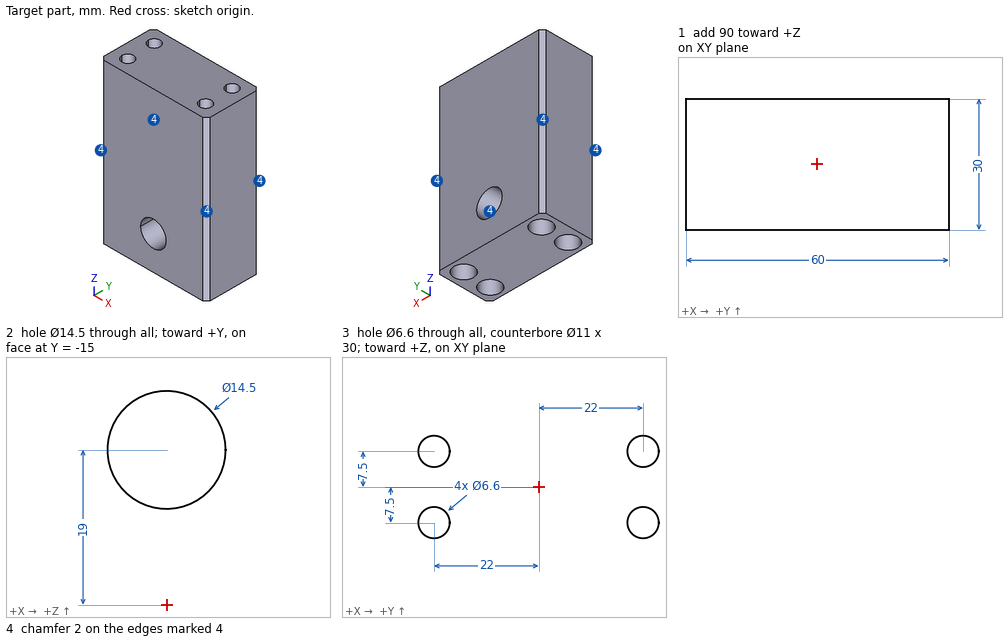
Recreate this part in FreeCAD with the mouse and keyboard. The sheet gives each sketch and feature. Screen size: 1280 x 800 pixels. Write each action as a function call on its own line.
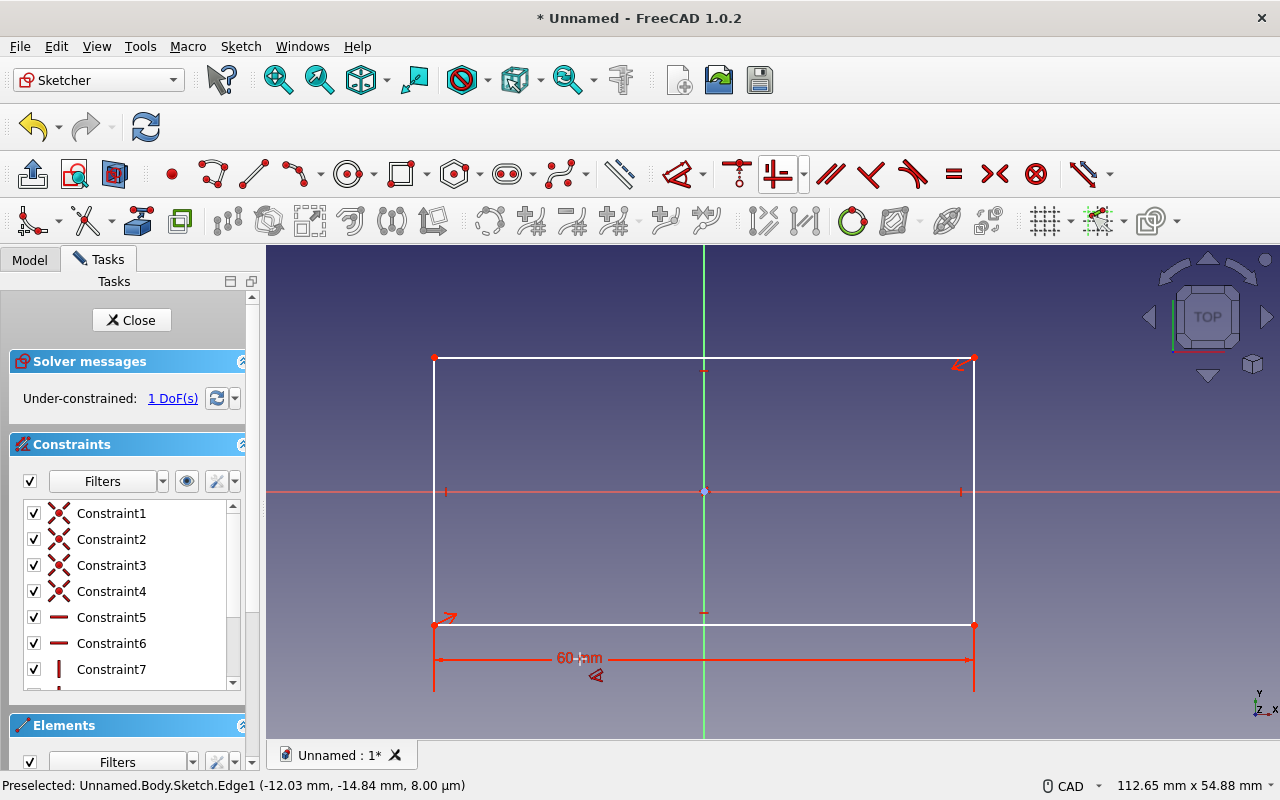
click(974, 545)
click(1008, 430)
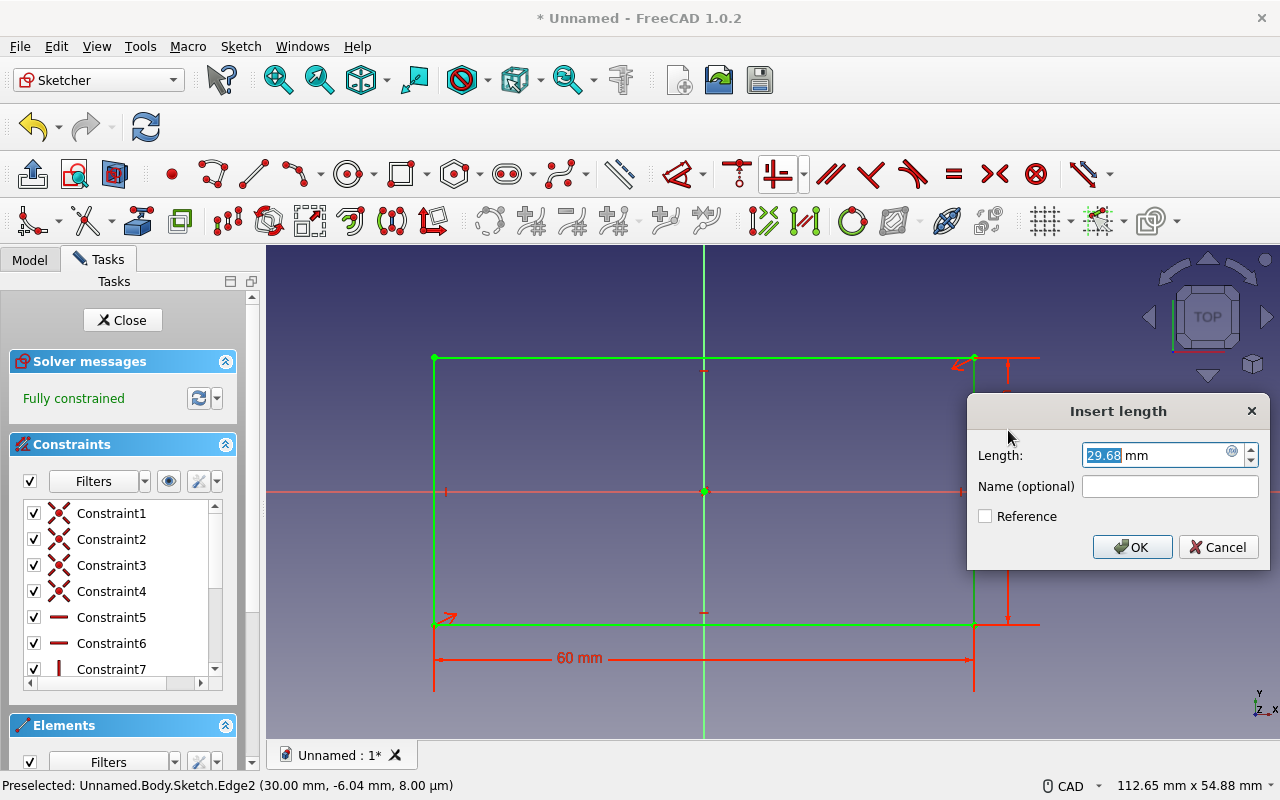
text(30)
key(Return)
key(Escape)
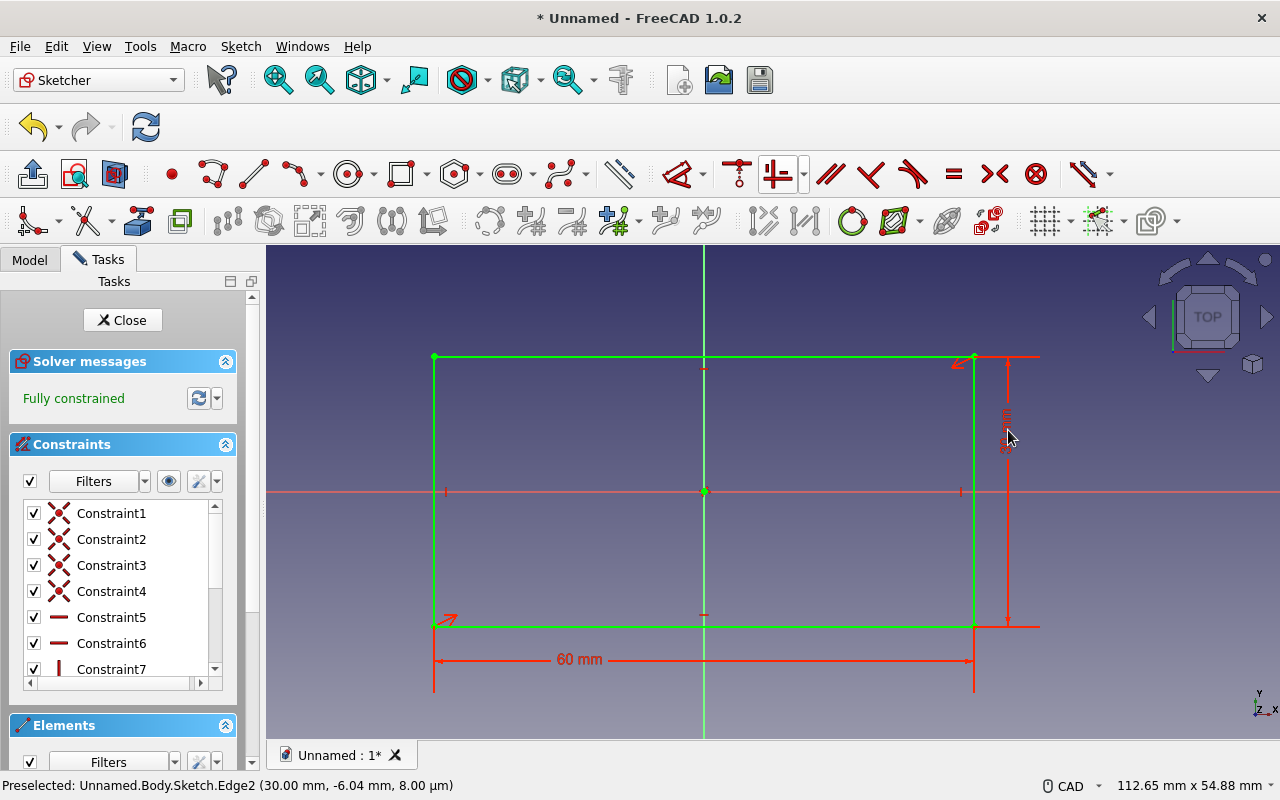
click(123, 320)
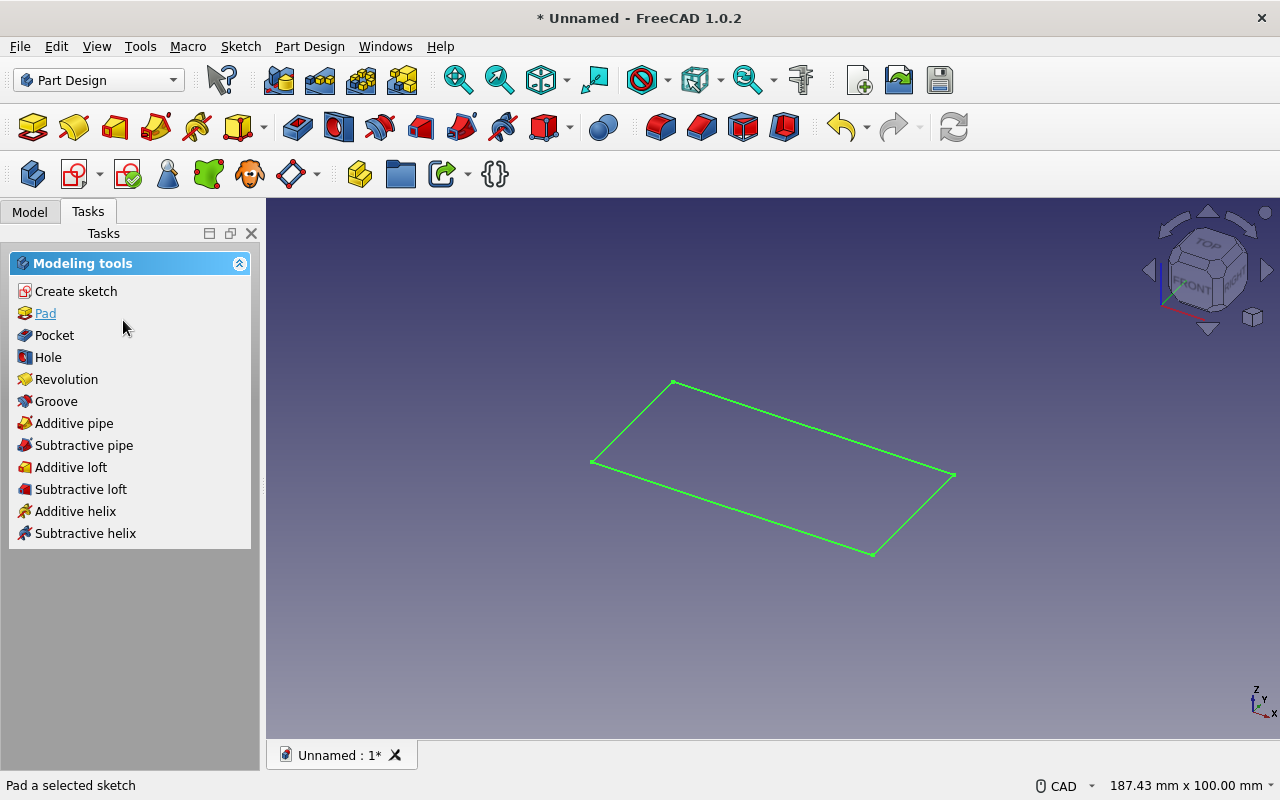
click(33, 128)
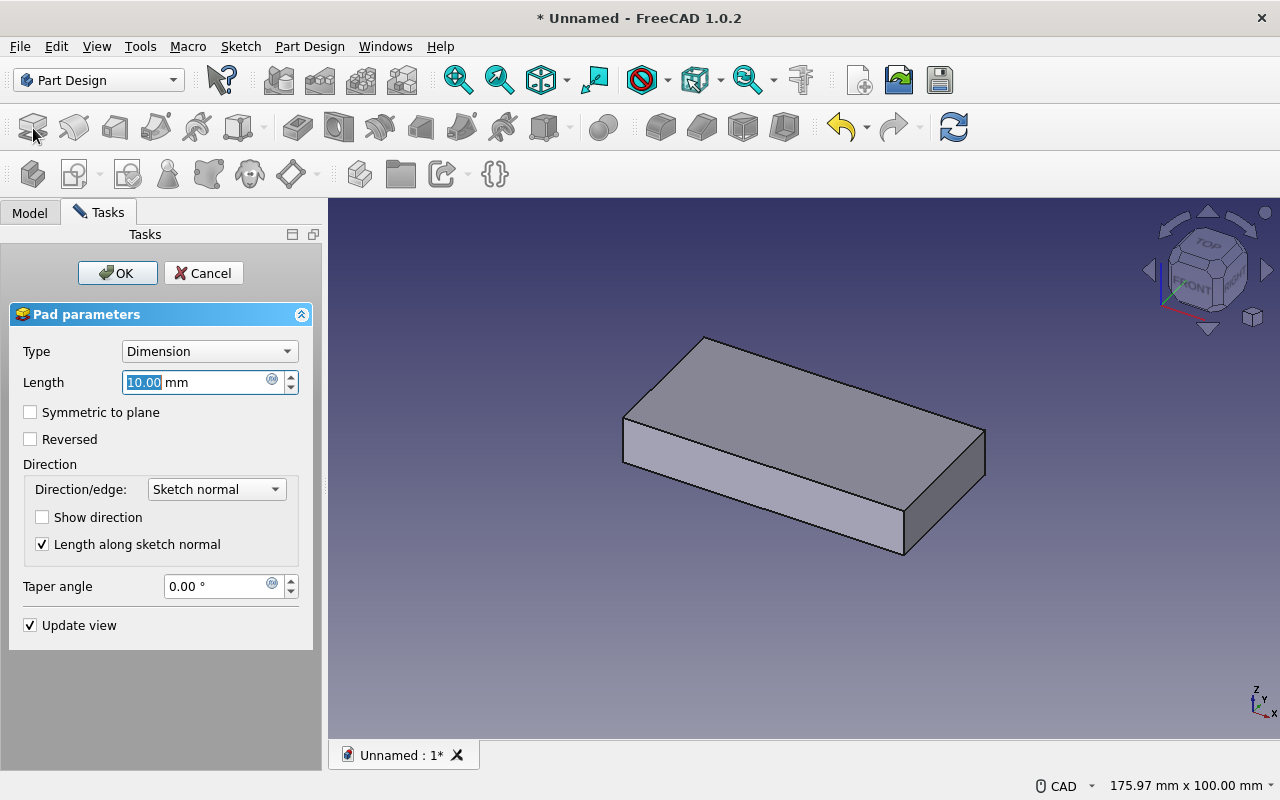
text(90)
key(Tab)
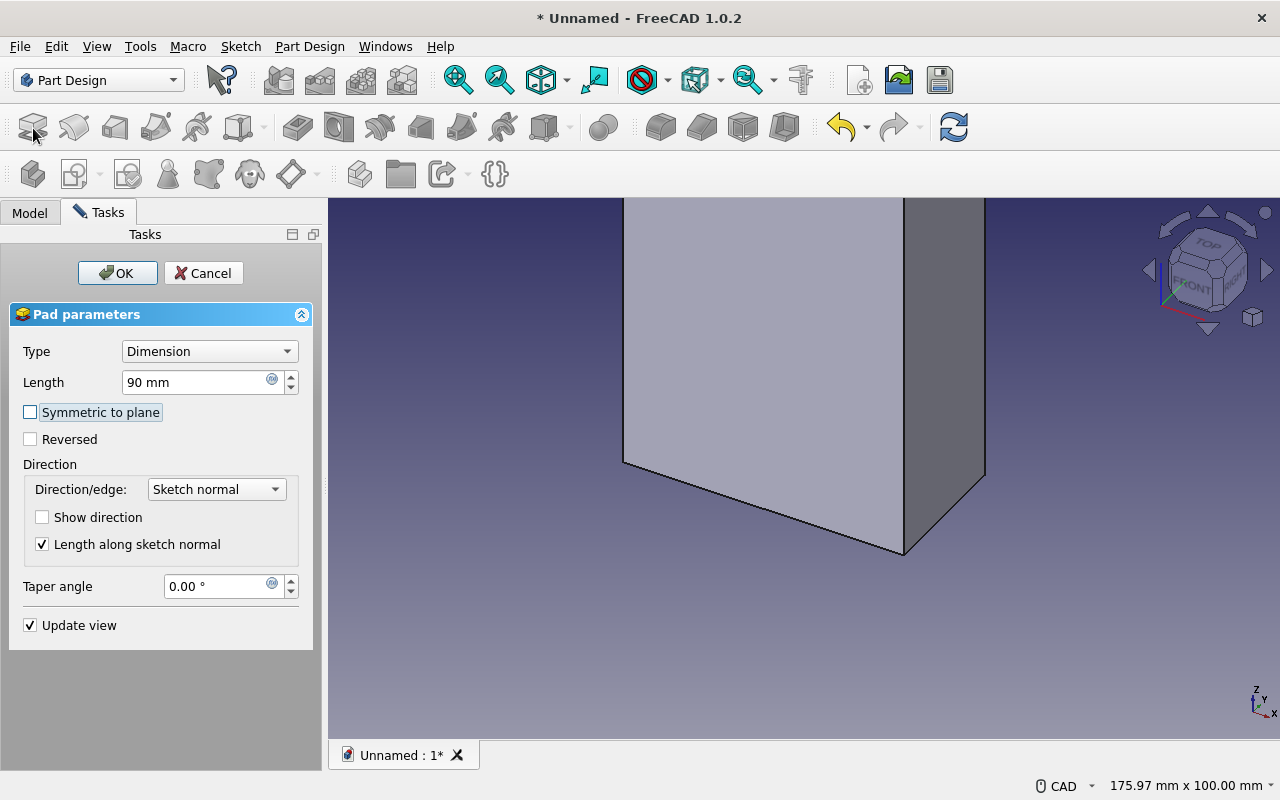
click(118, 273)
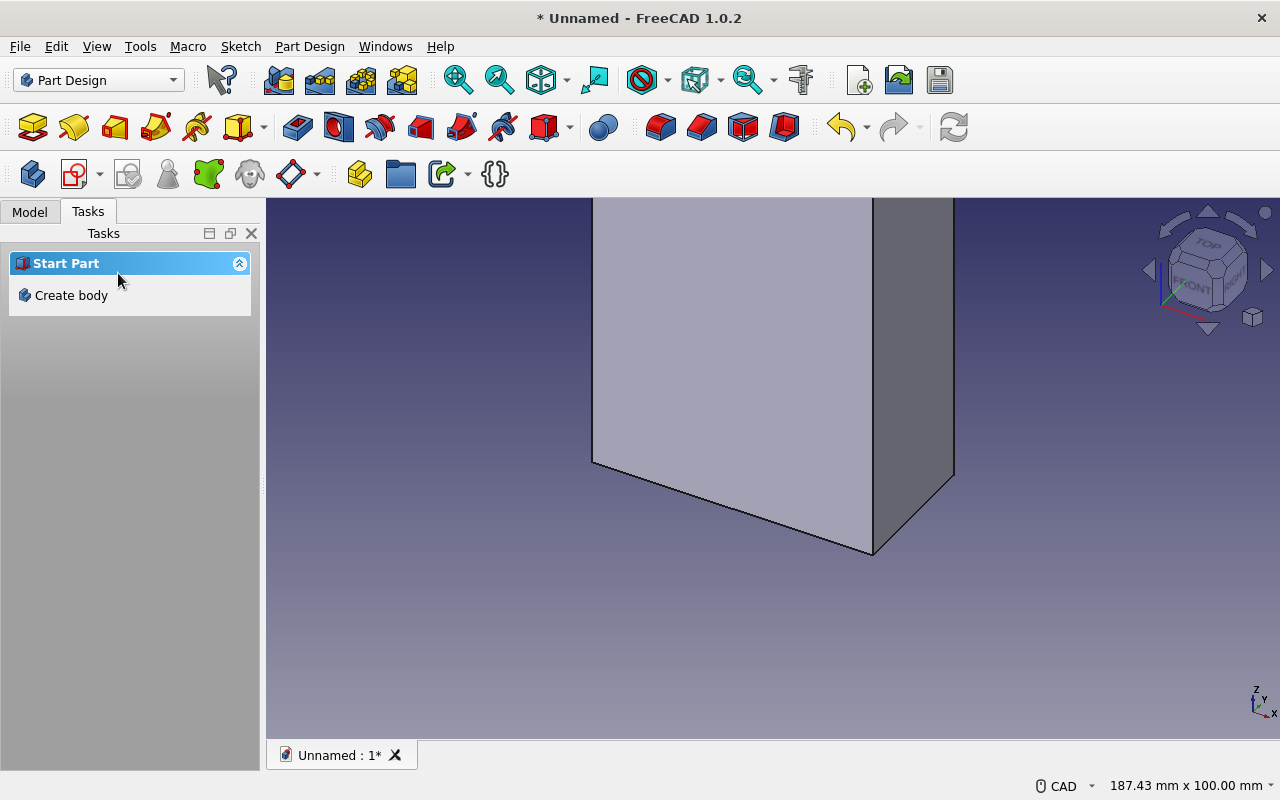
click(459, 80)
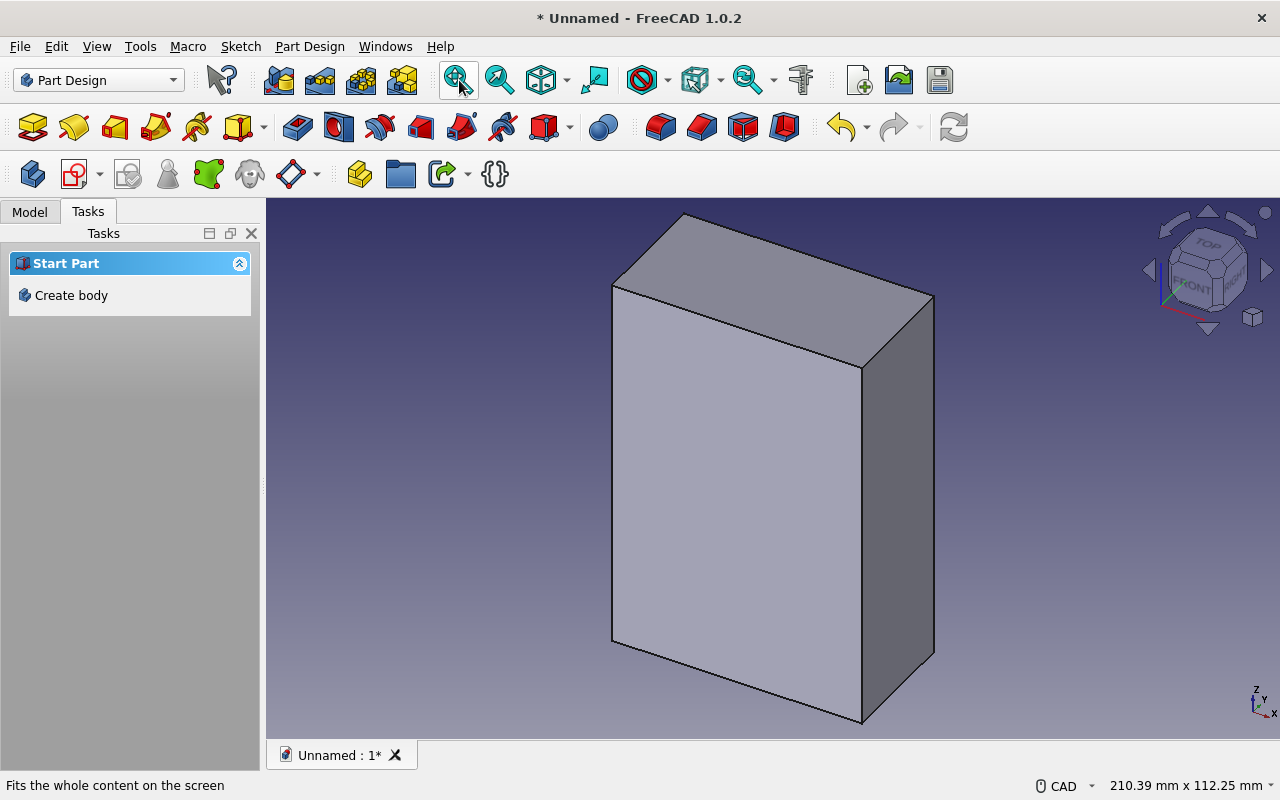
click(737, 453)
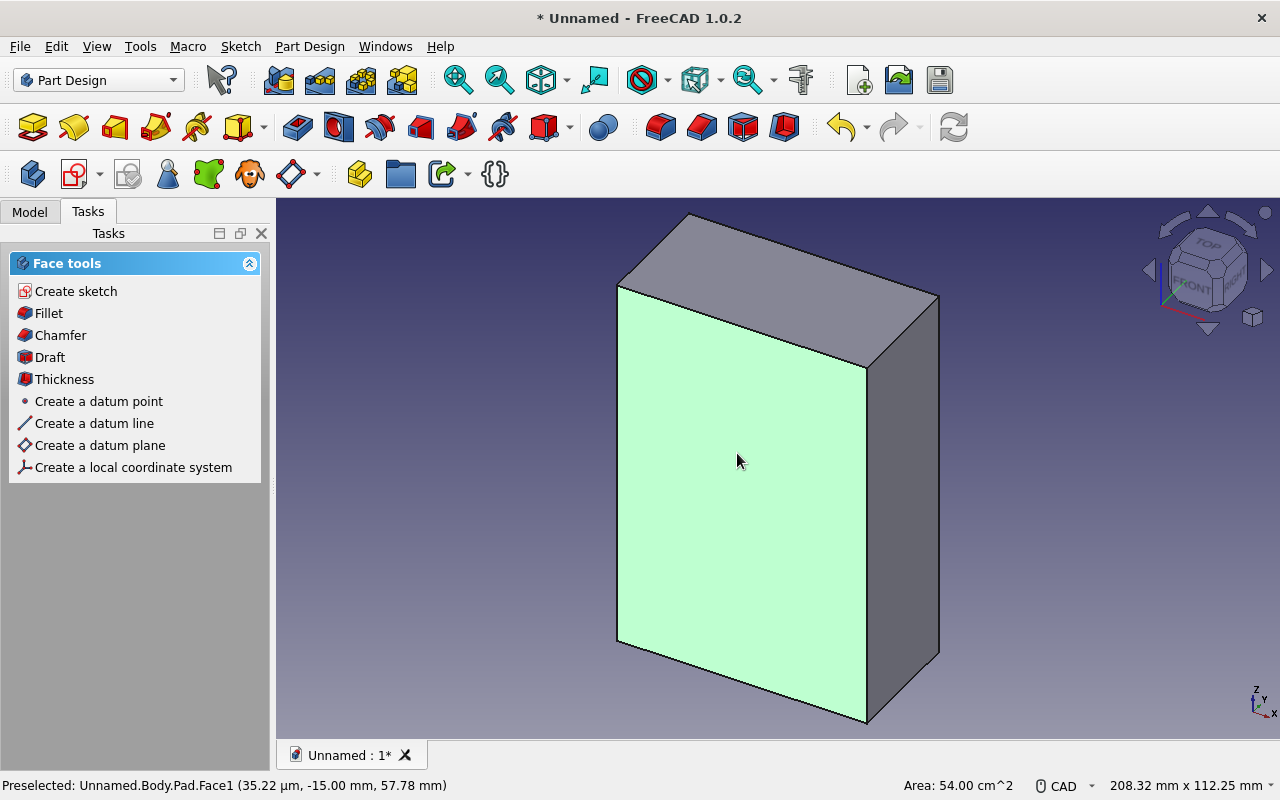
click(74, 174)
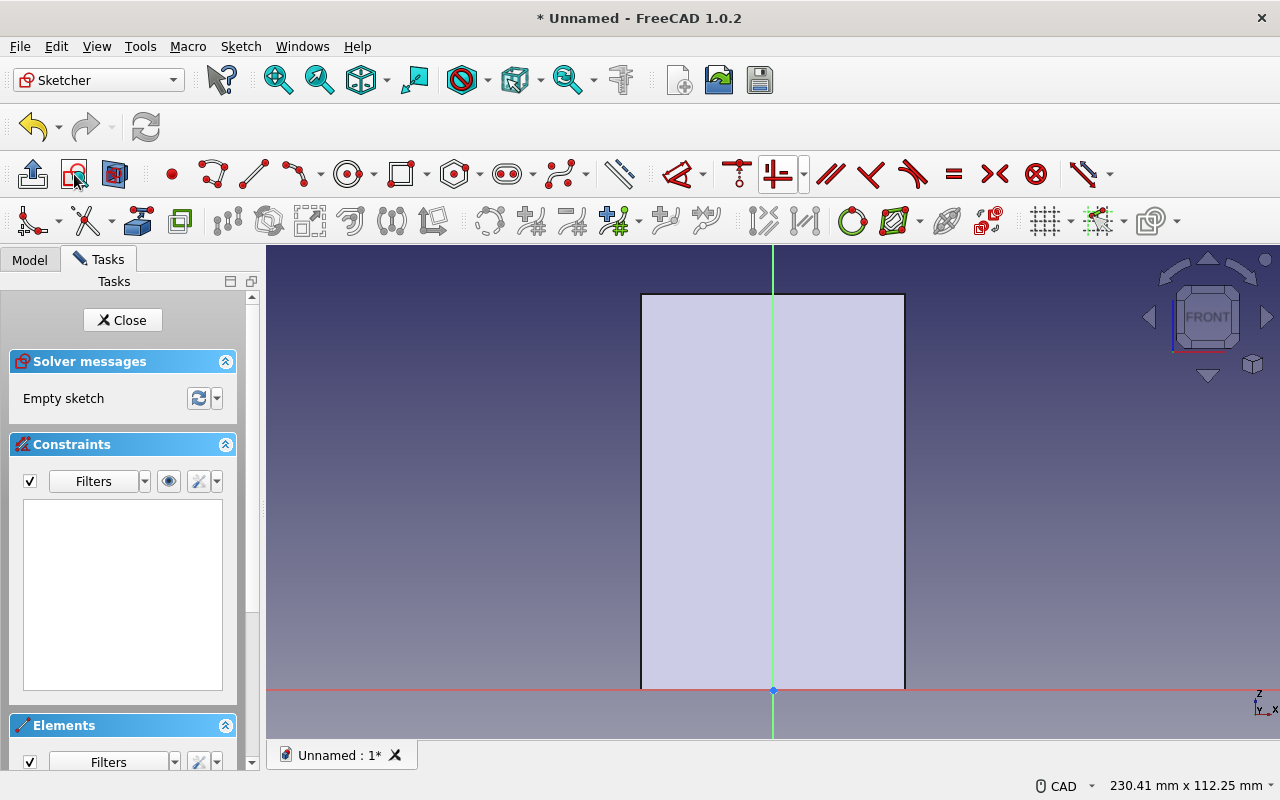
scroll(813, 711, up, 5)